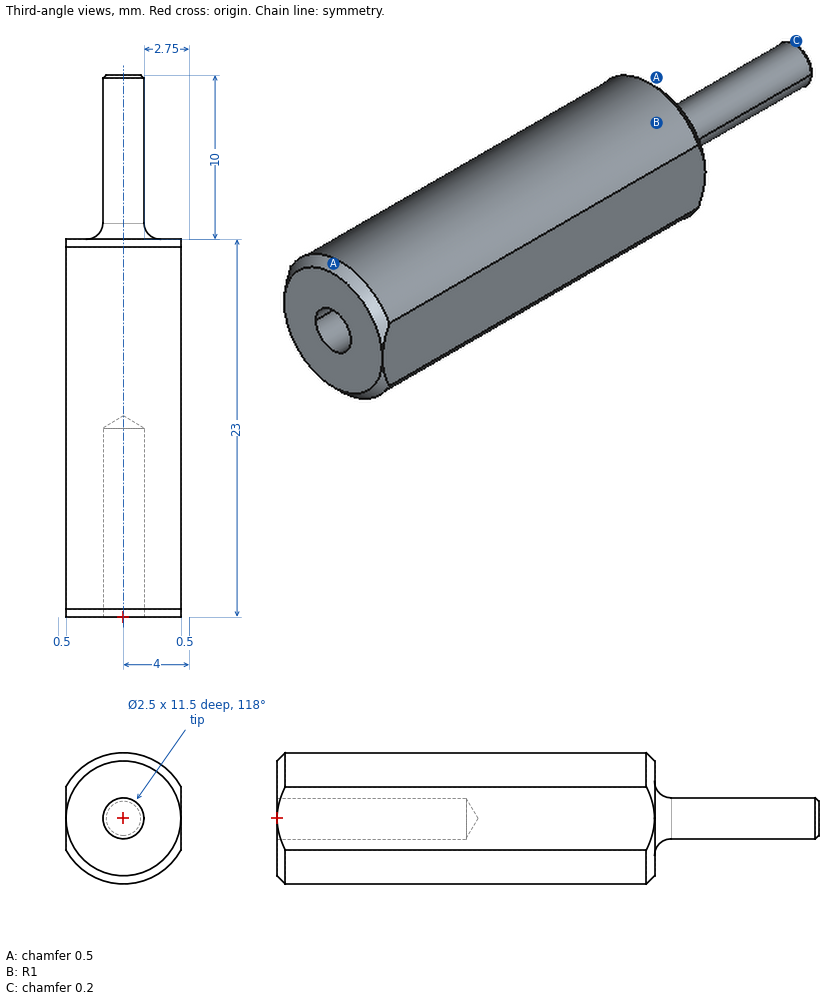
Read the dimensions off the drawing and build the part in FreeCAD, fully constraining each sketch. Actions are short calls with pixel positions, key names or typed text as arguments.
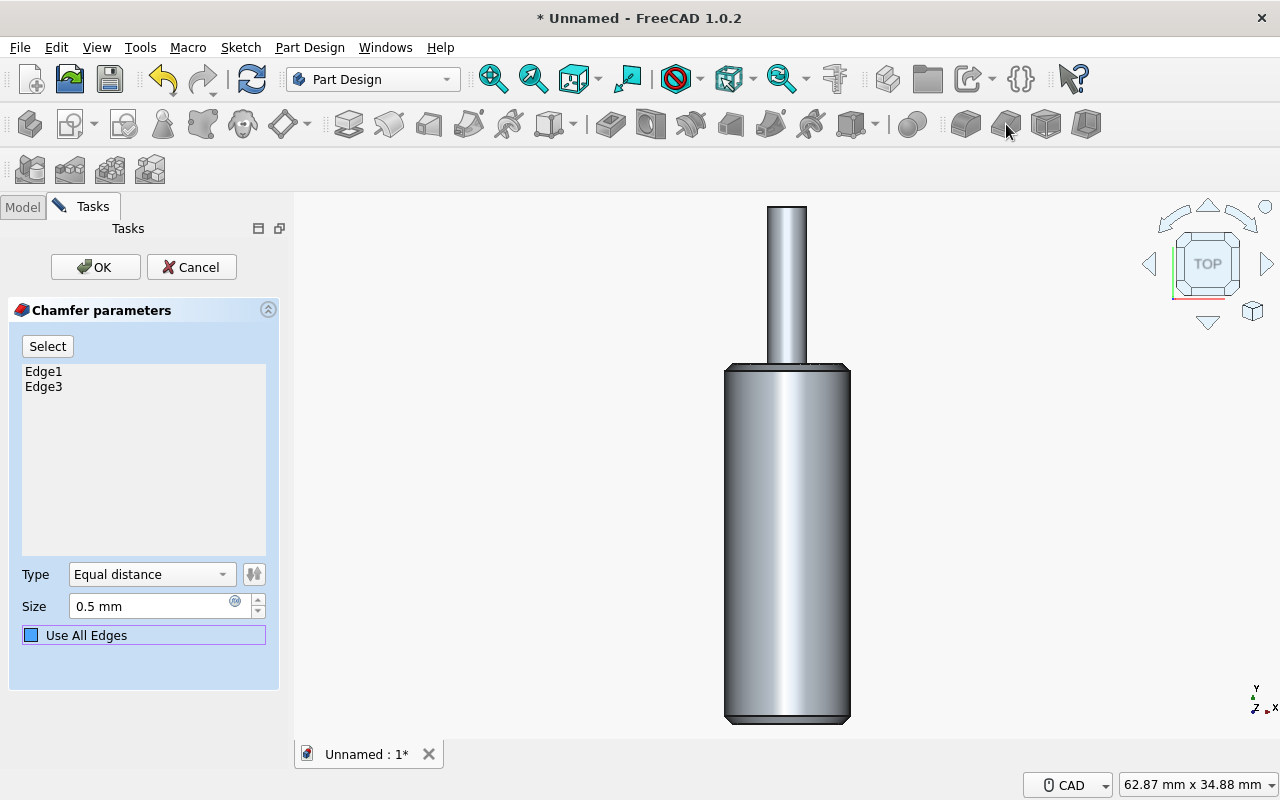
click(96, 267)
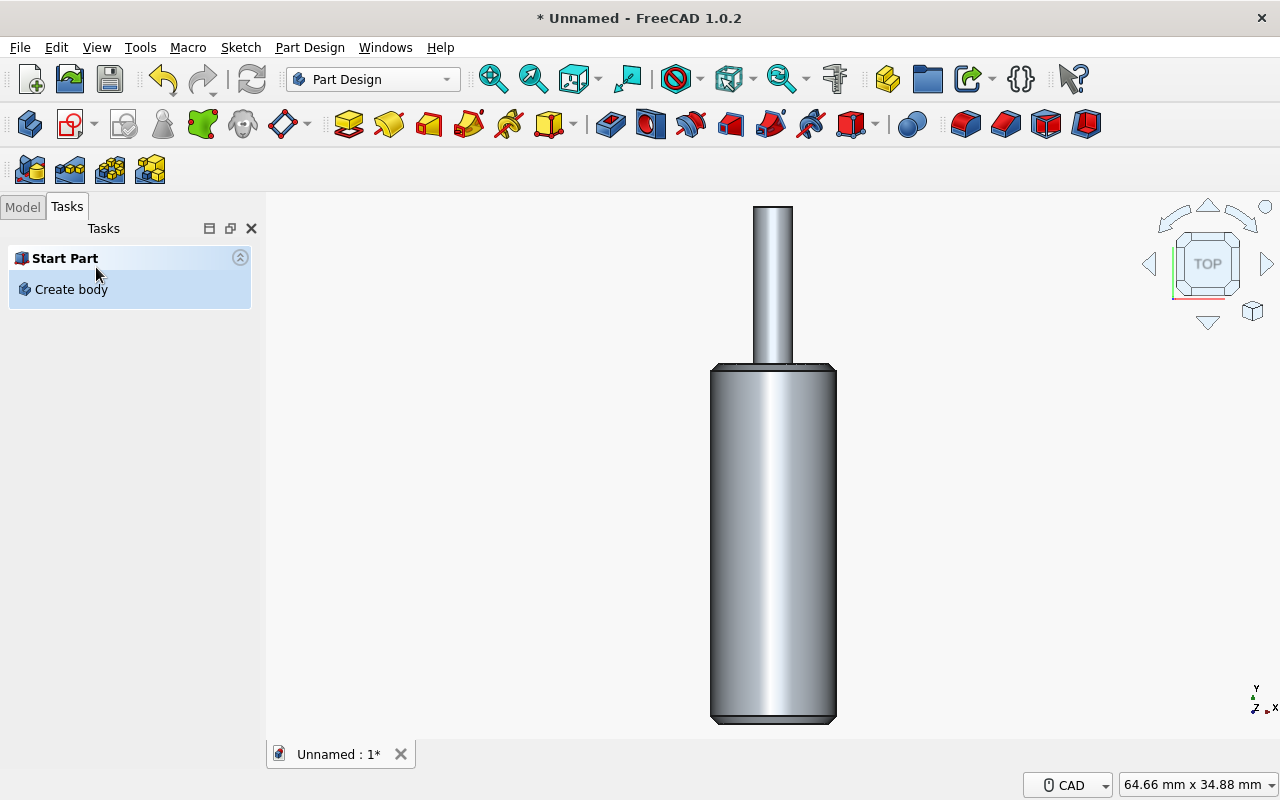
key(0)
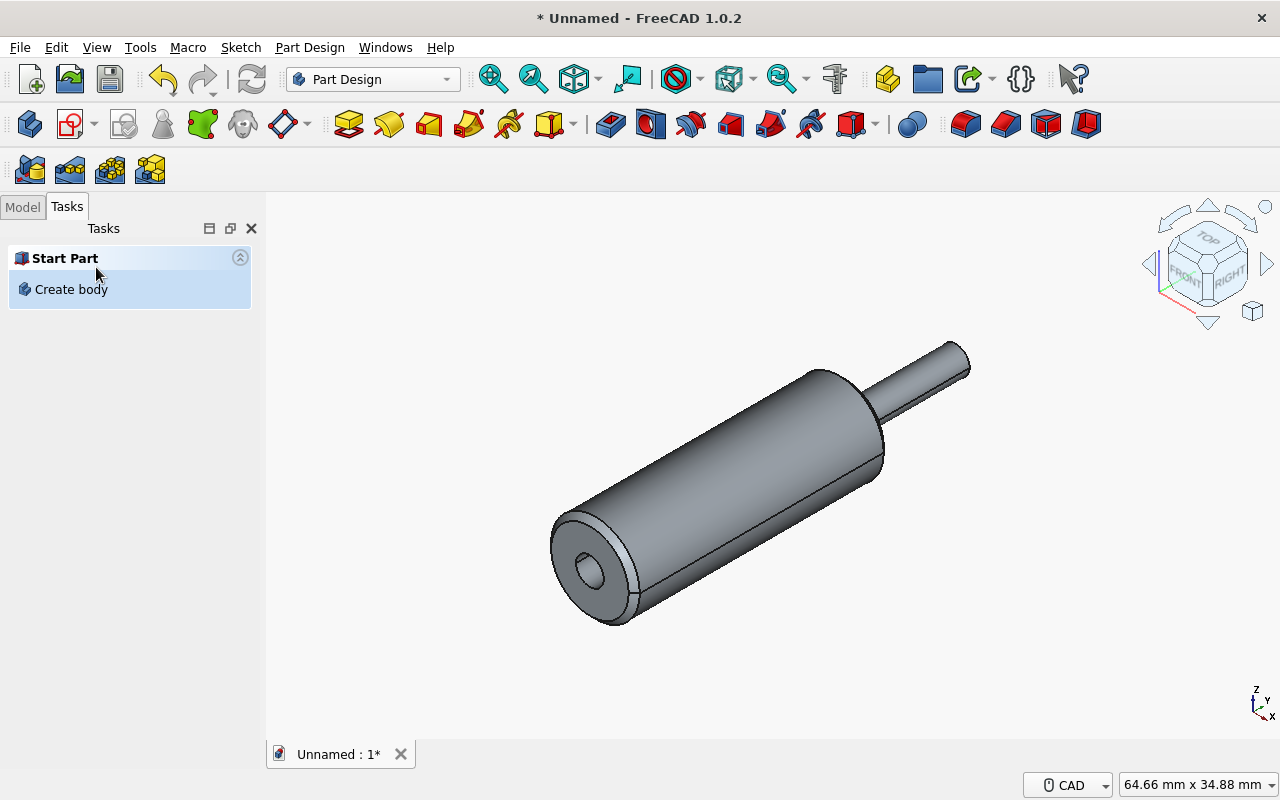
key(2)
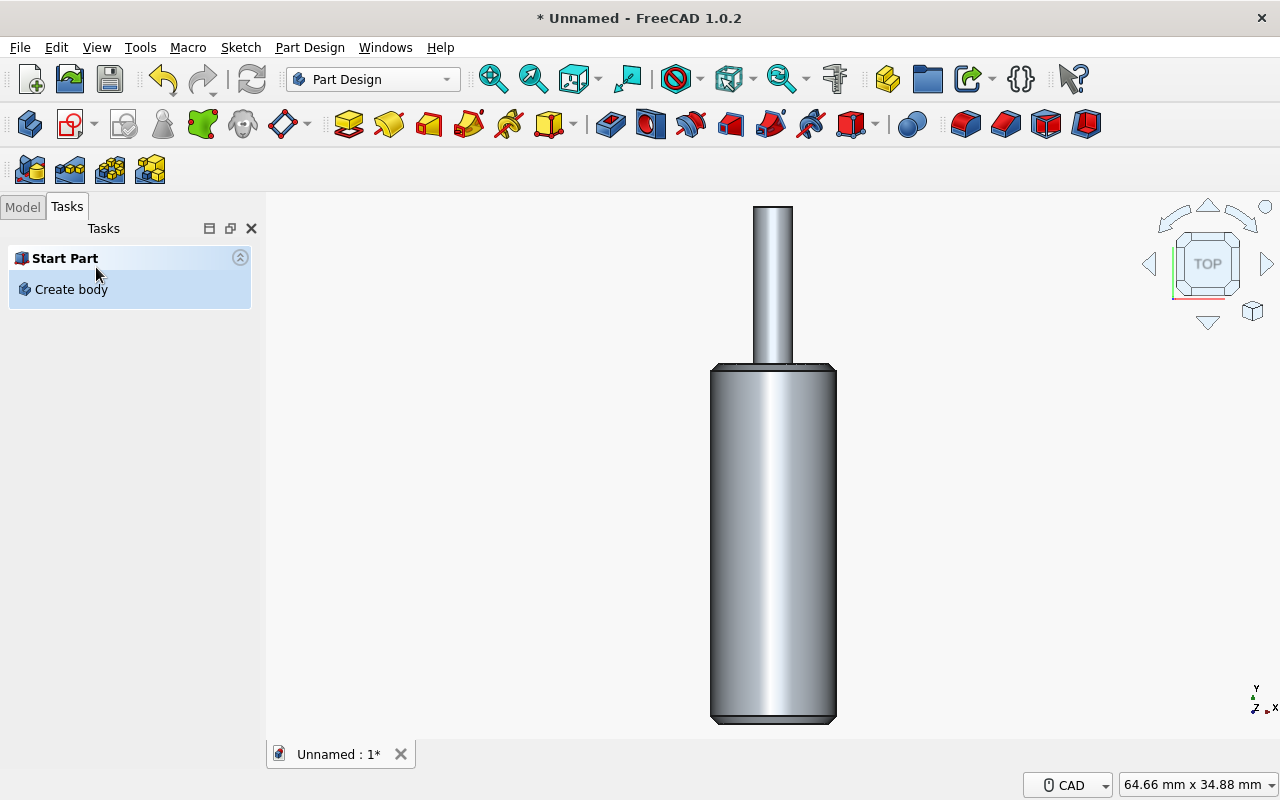
key(1)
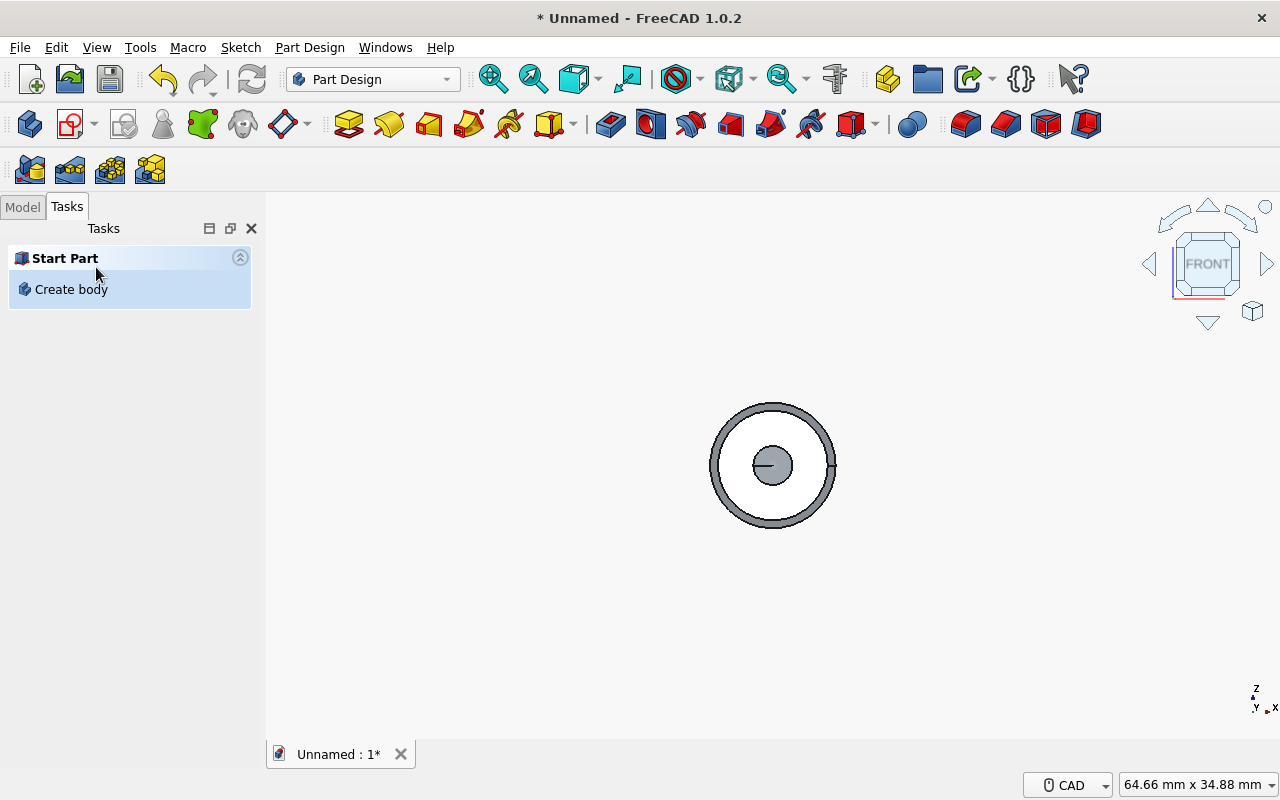
key(v)
key(f)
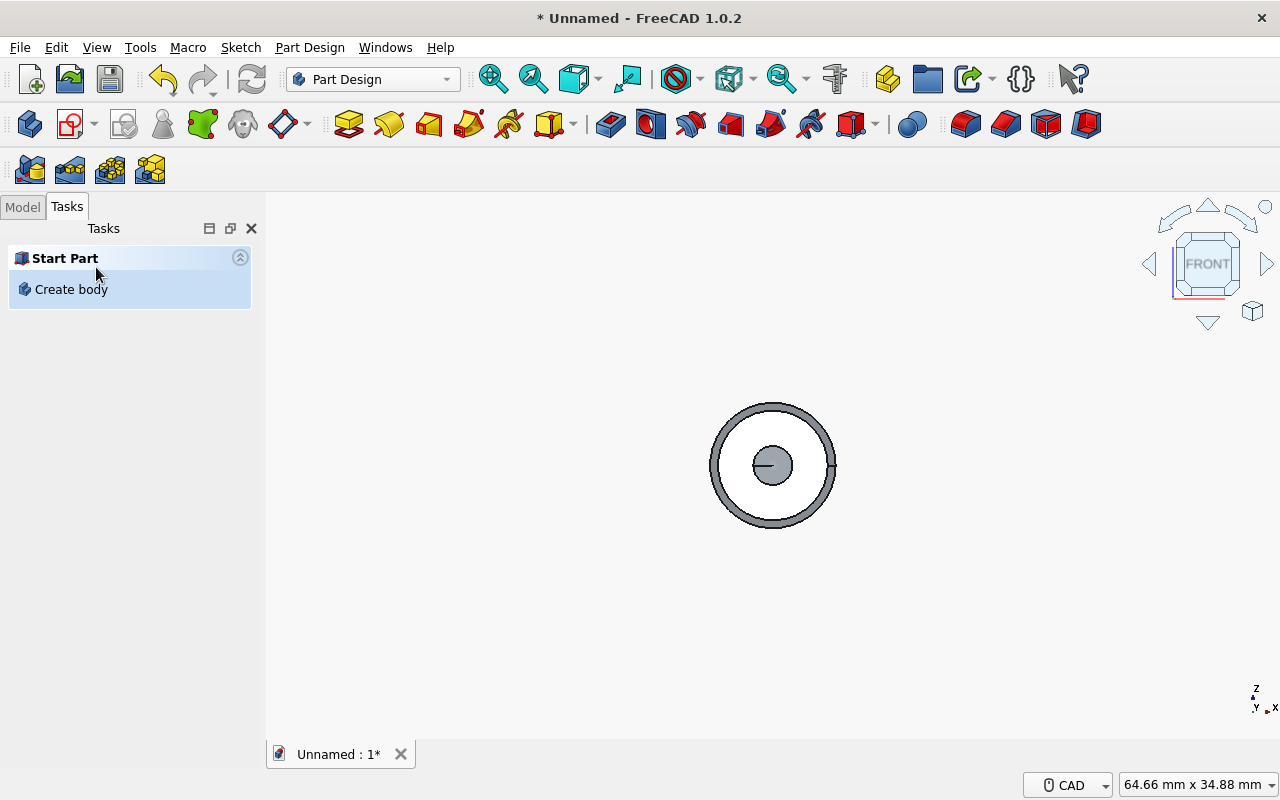
key(3)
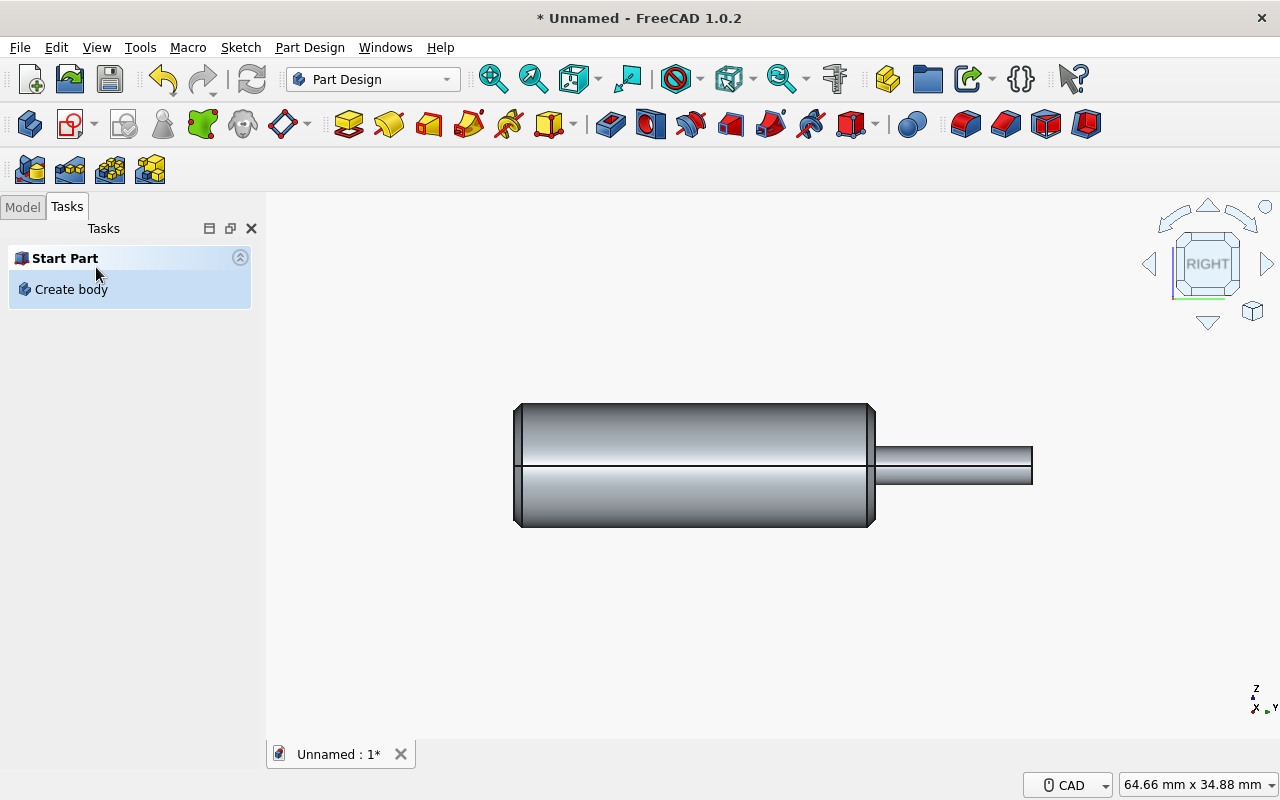
key(5)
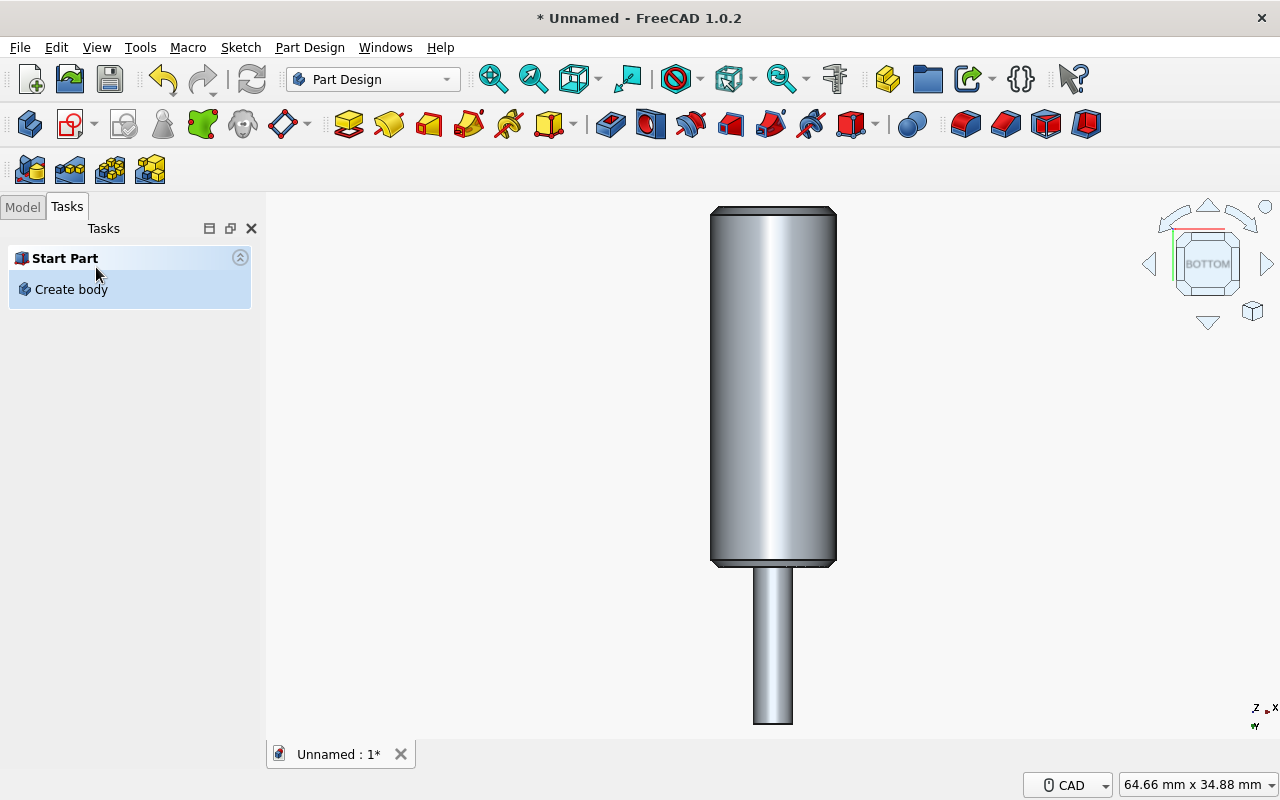
key(4)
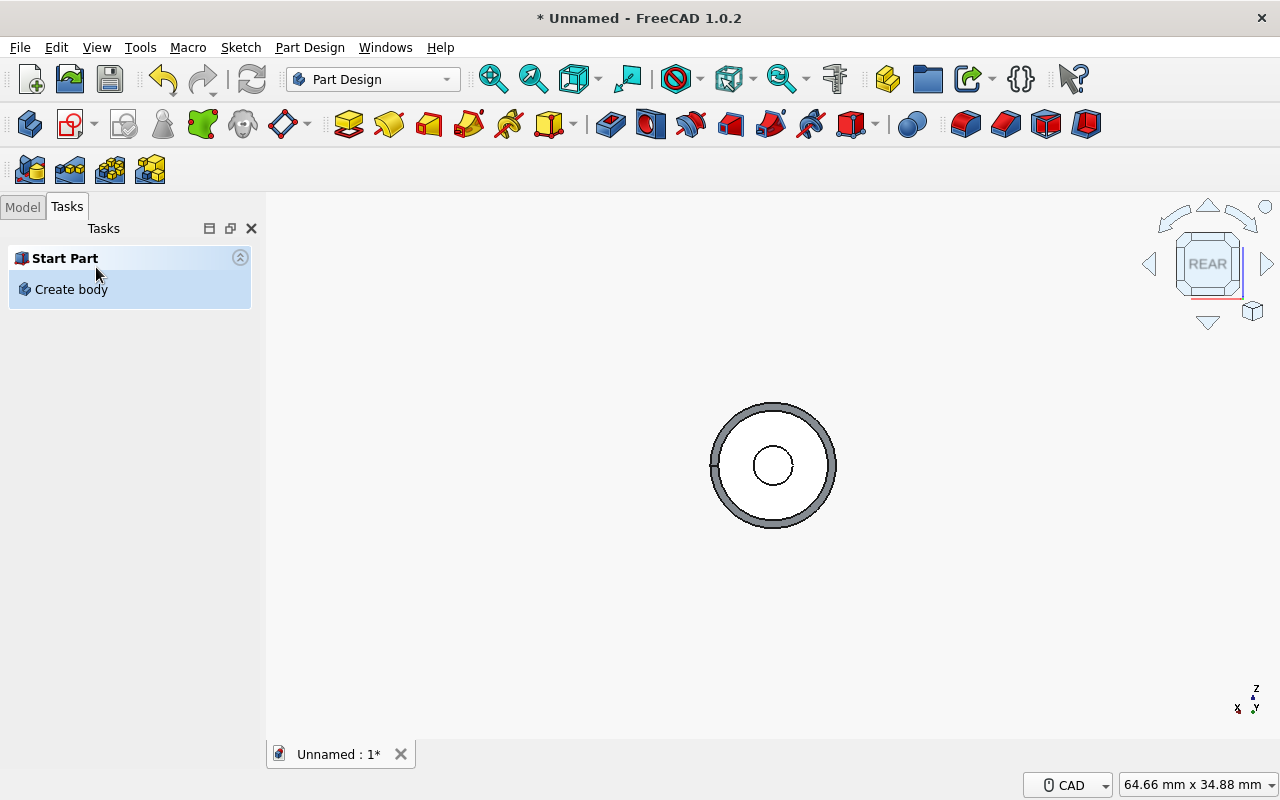
key(v)
key(f)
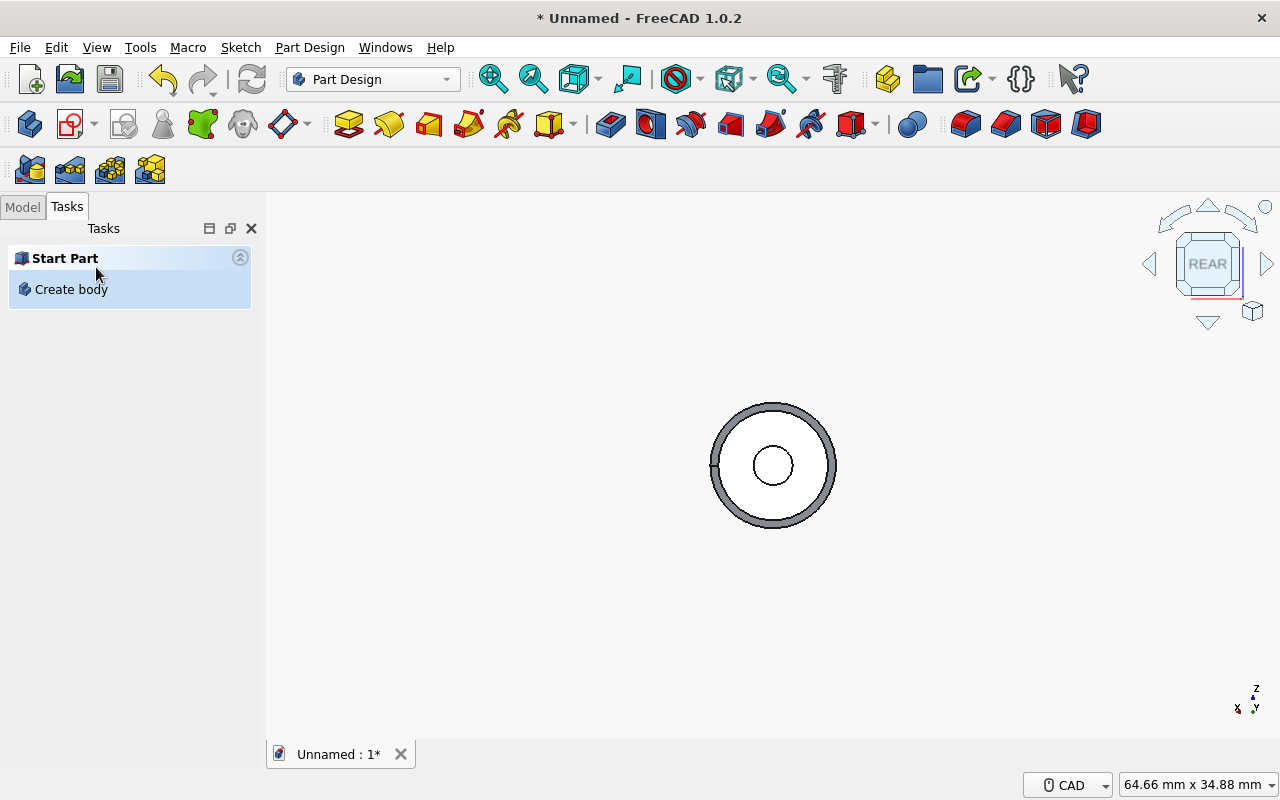
key(6)